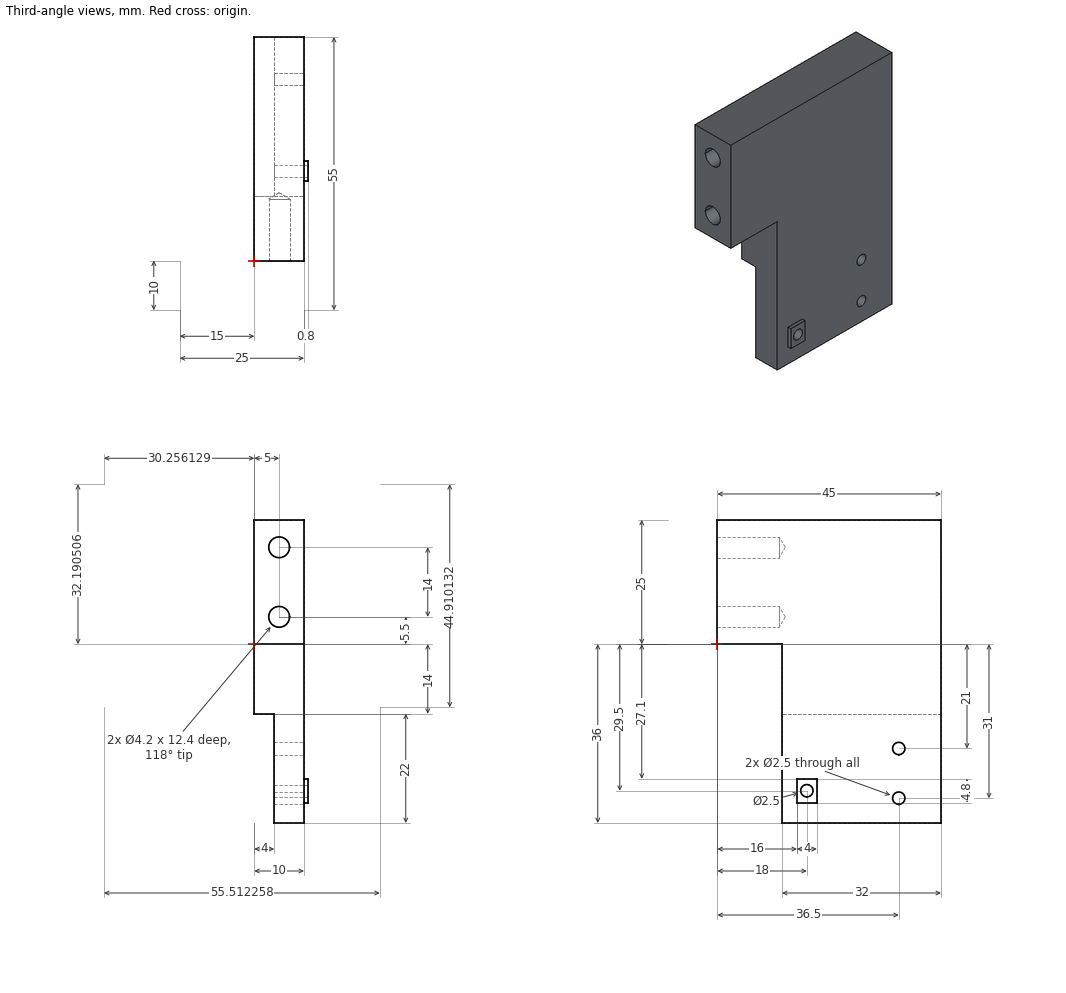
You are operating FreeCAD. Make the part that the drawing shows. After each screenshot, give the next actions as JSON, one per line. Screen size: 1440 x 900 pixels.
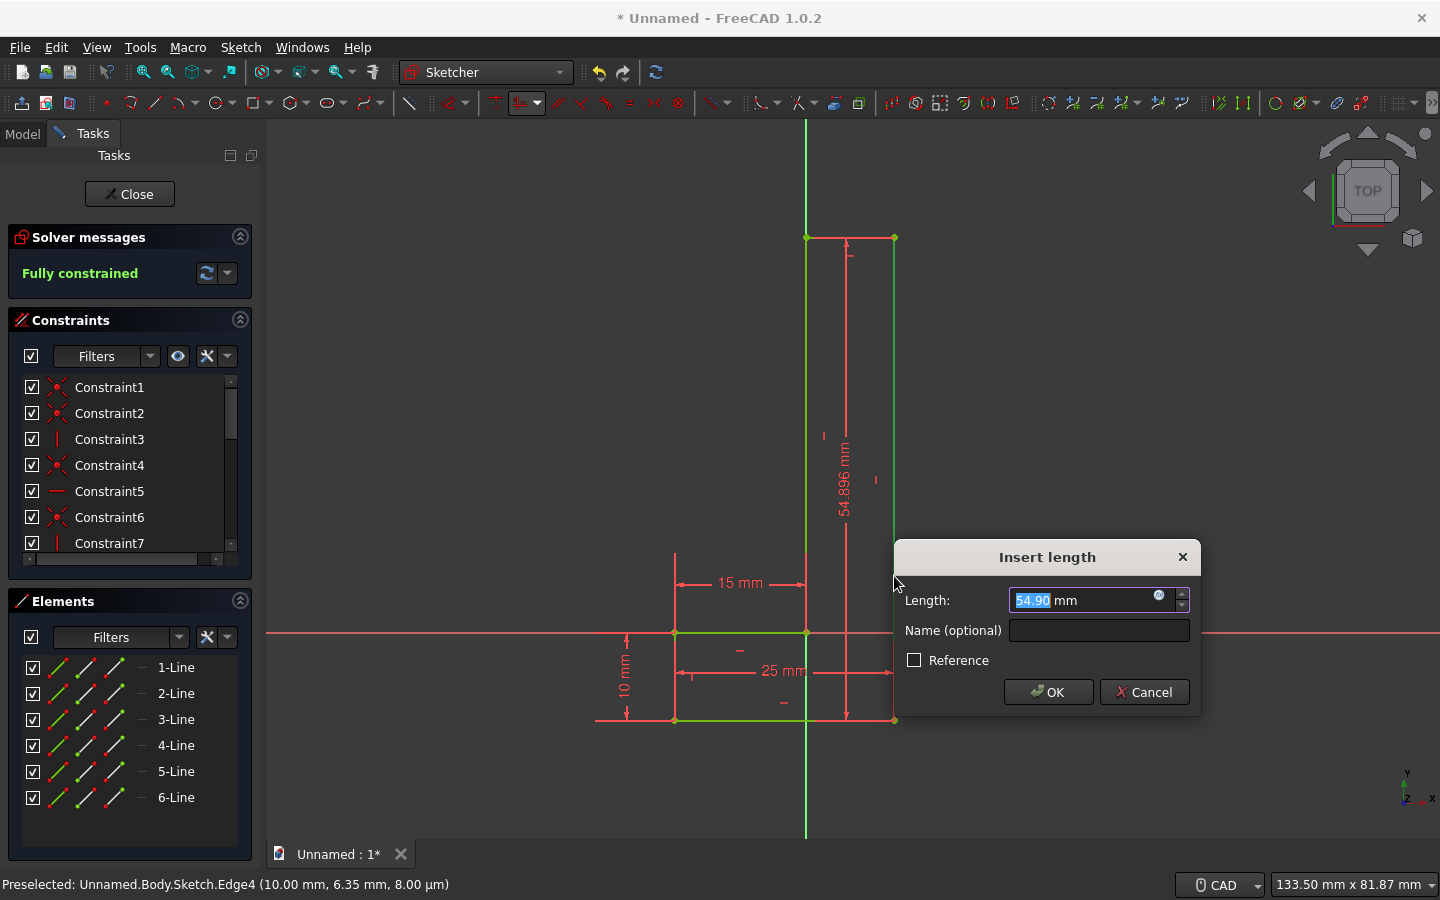
{"action": "type", "text": "55"}
{"action": "key", "text": "Return"}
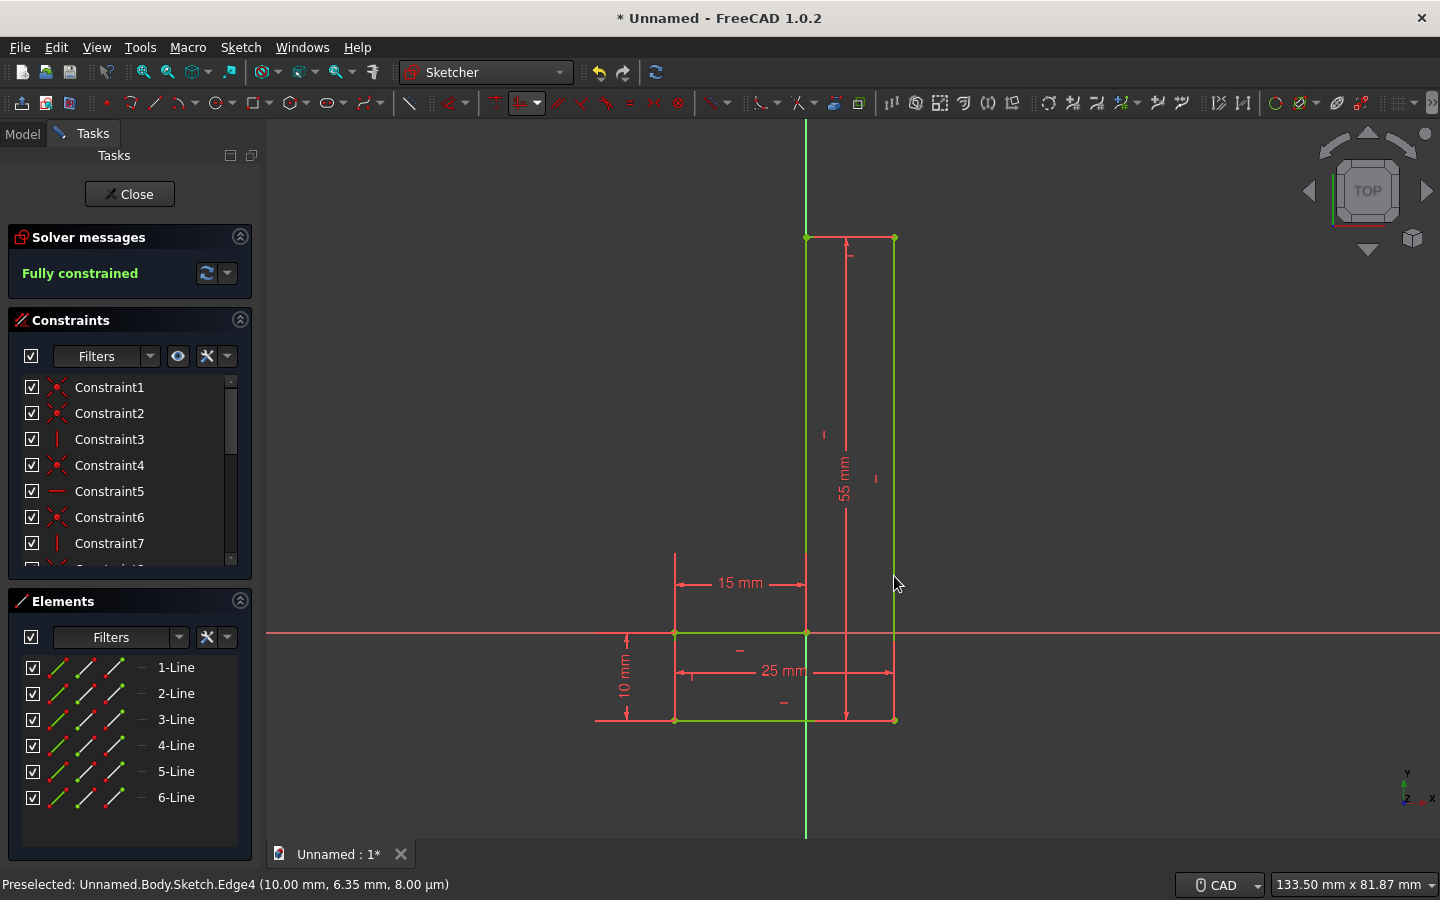
{"action": "left_click", "coordinate": [130, 194]}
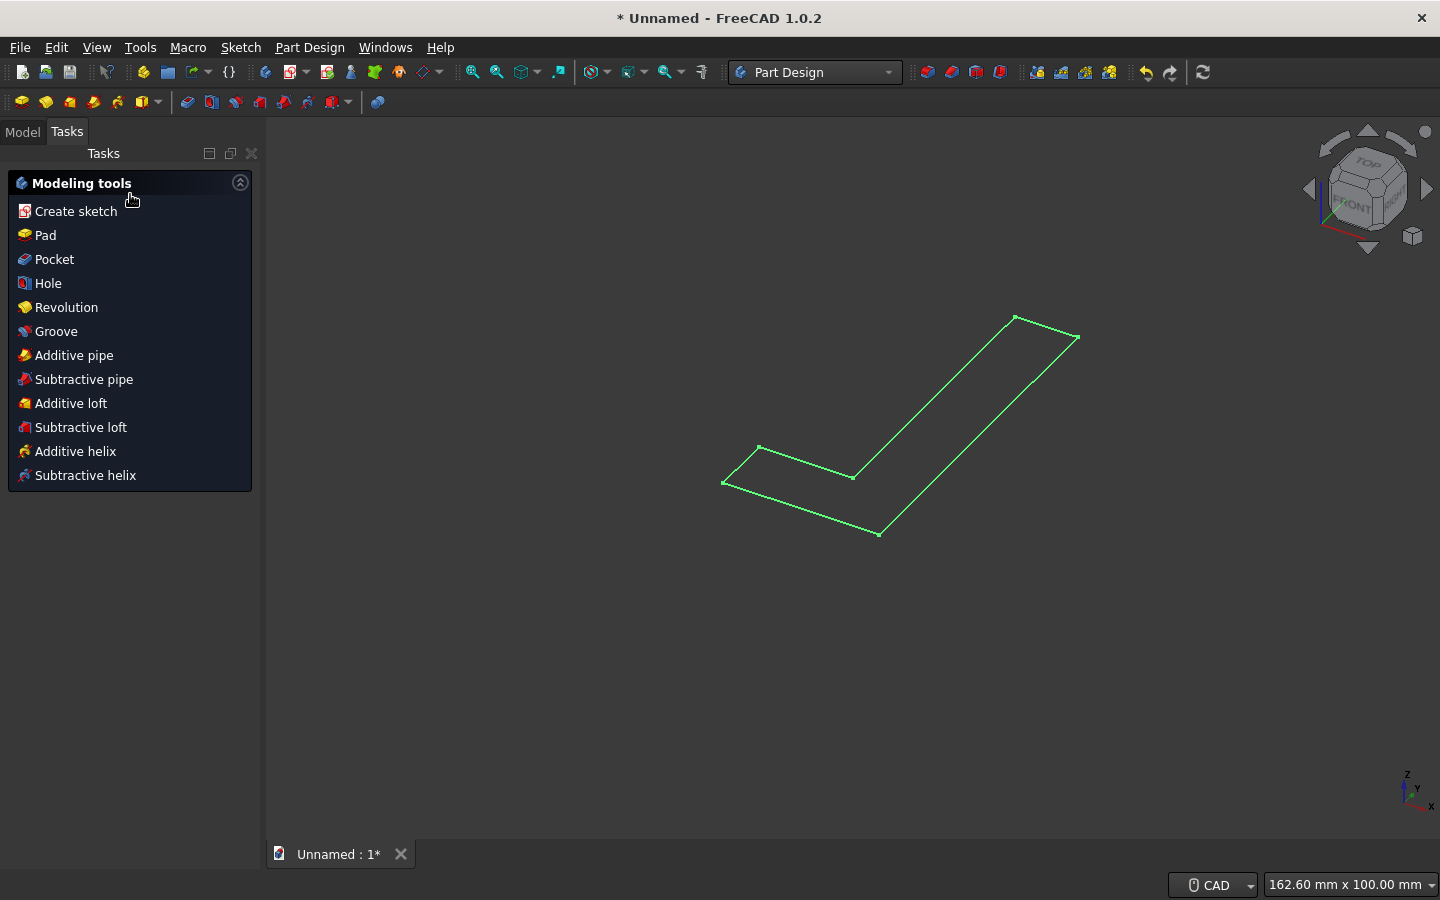
{"action": "left_click", "coordinate": [22, 102]}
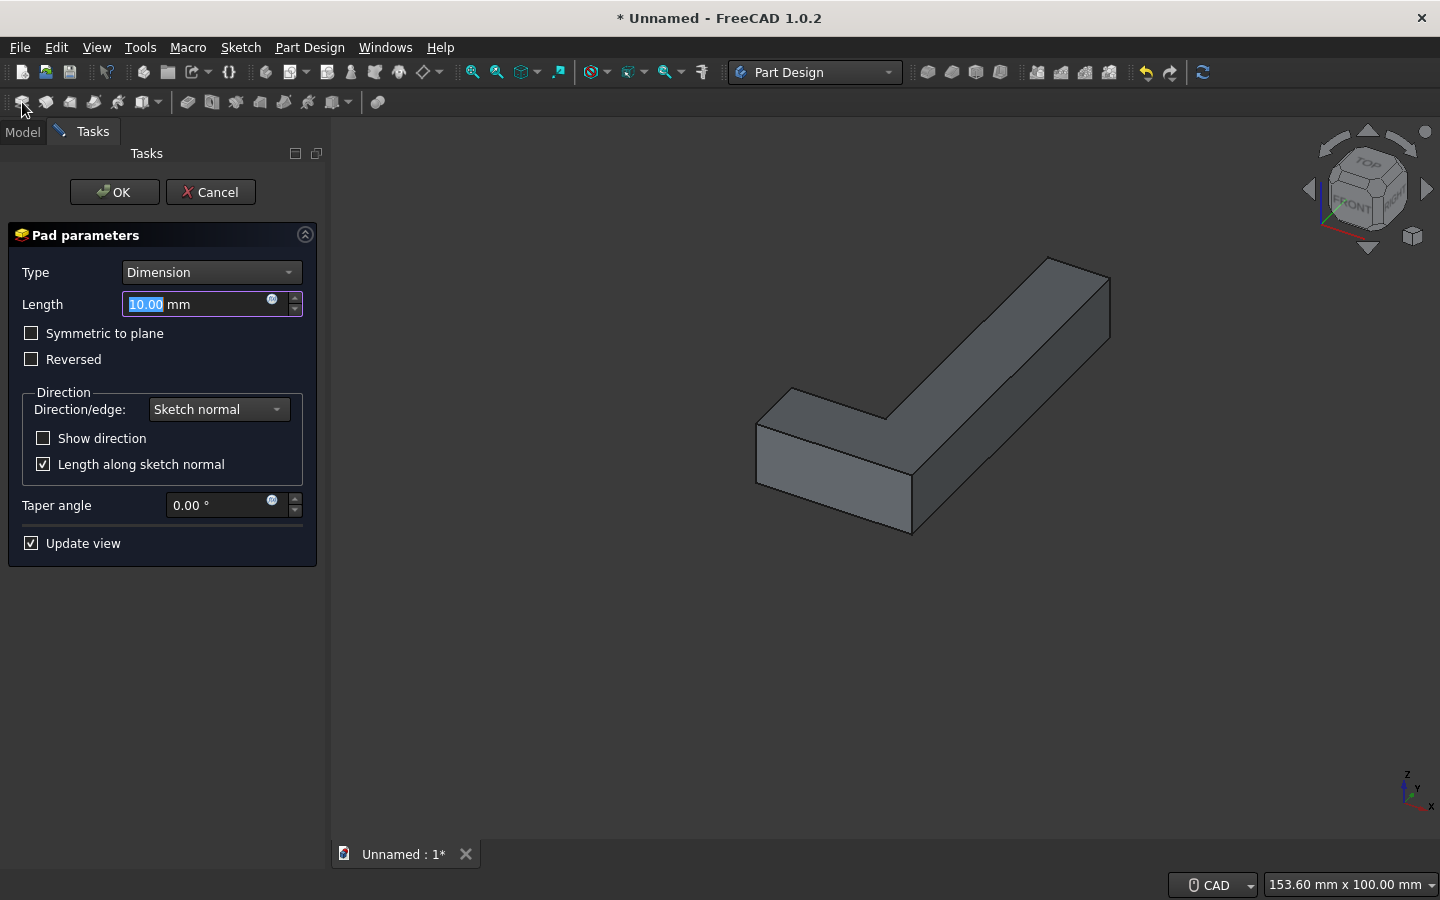
{"action": "type", "text": "25"}
{"action": "key", "text": "Tab"}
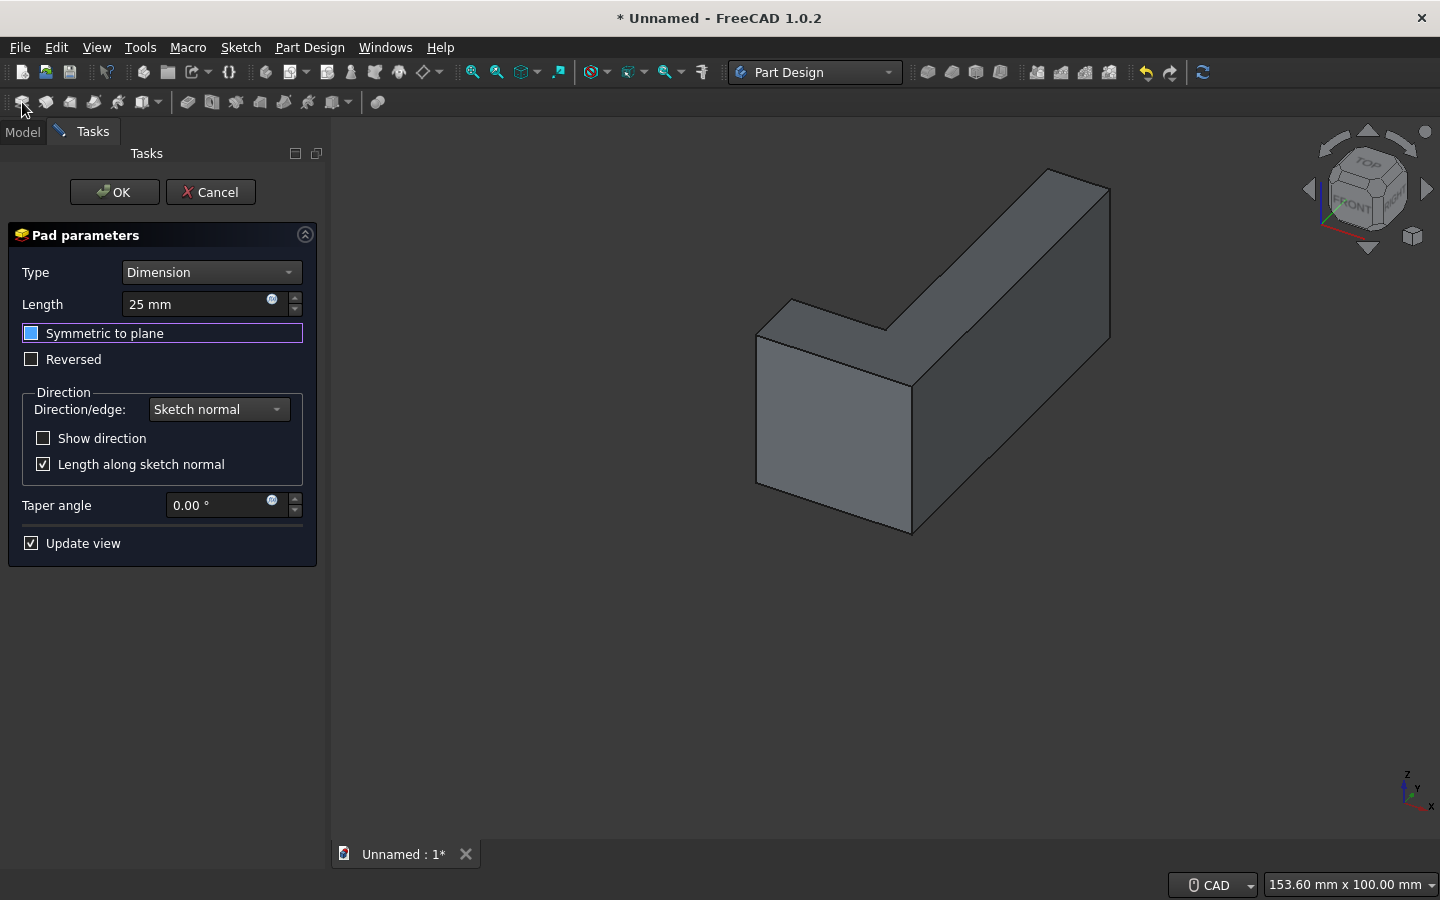
{"action": "left_click", "coordinate": [115, 192]}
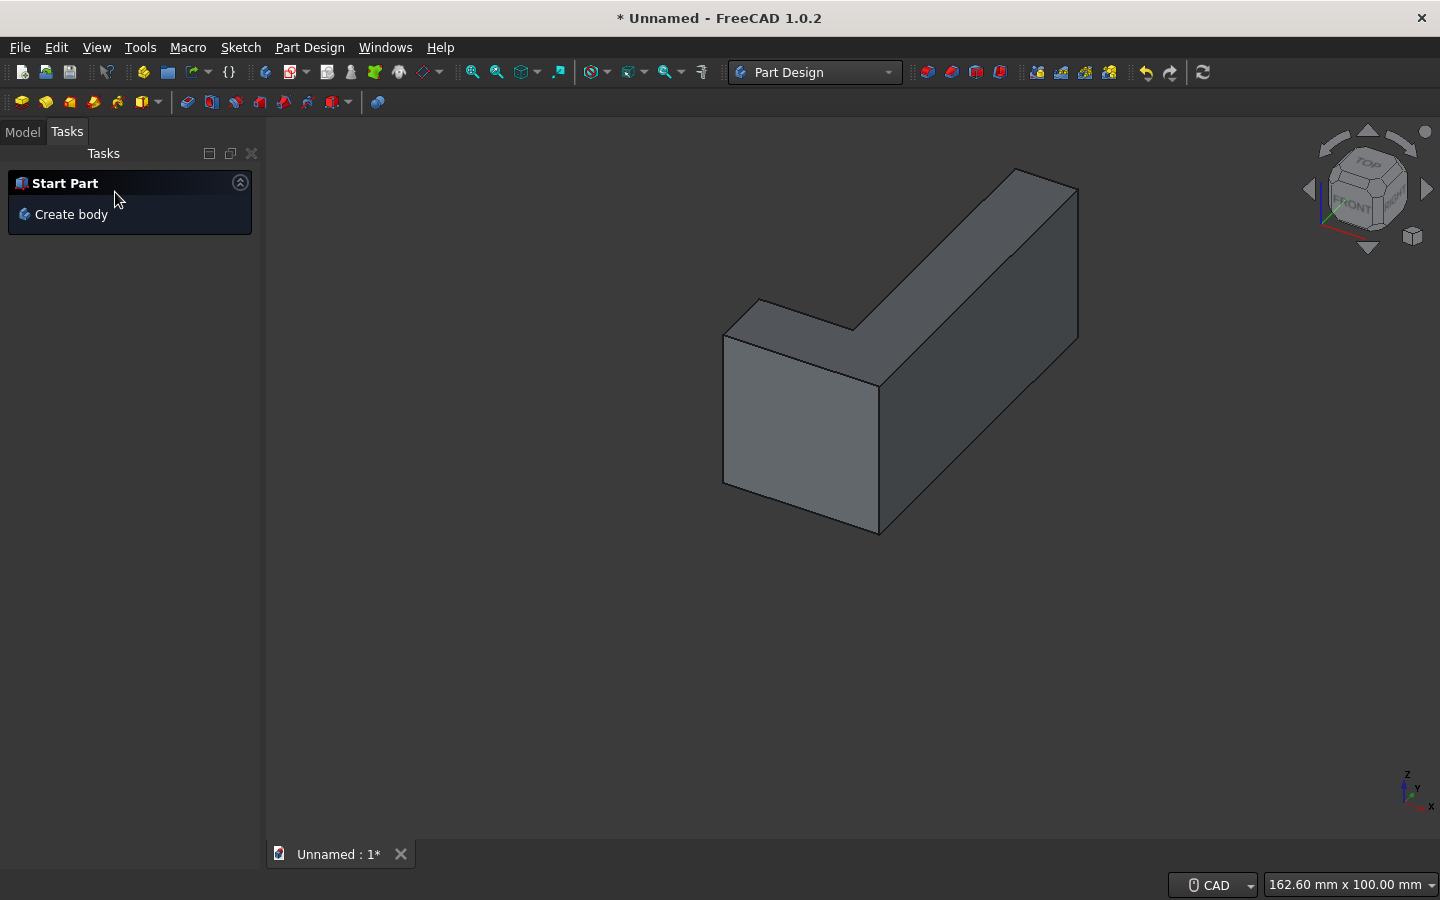
{"action": "key", "text": "6"}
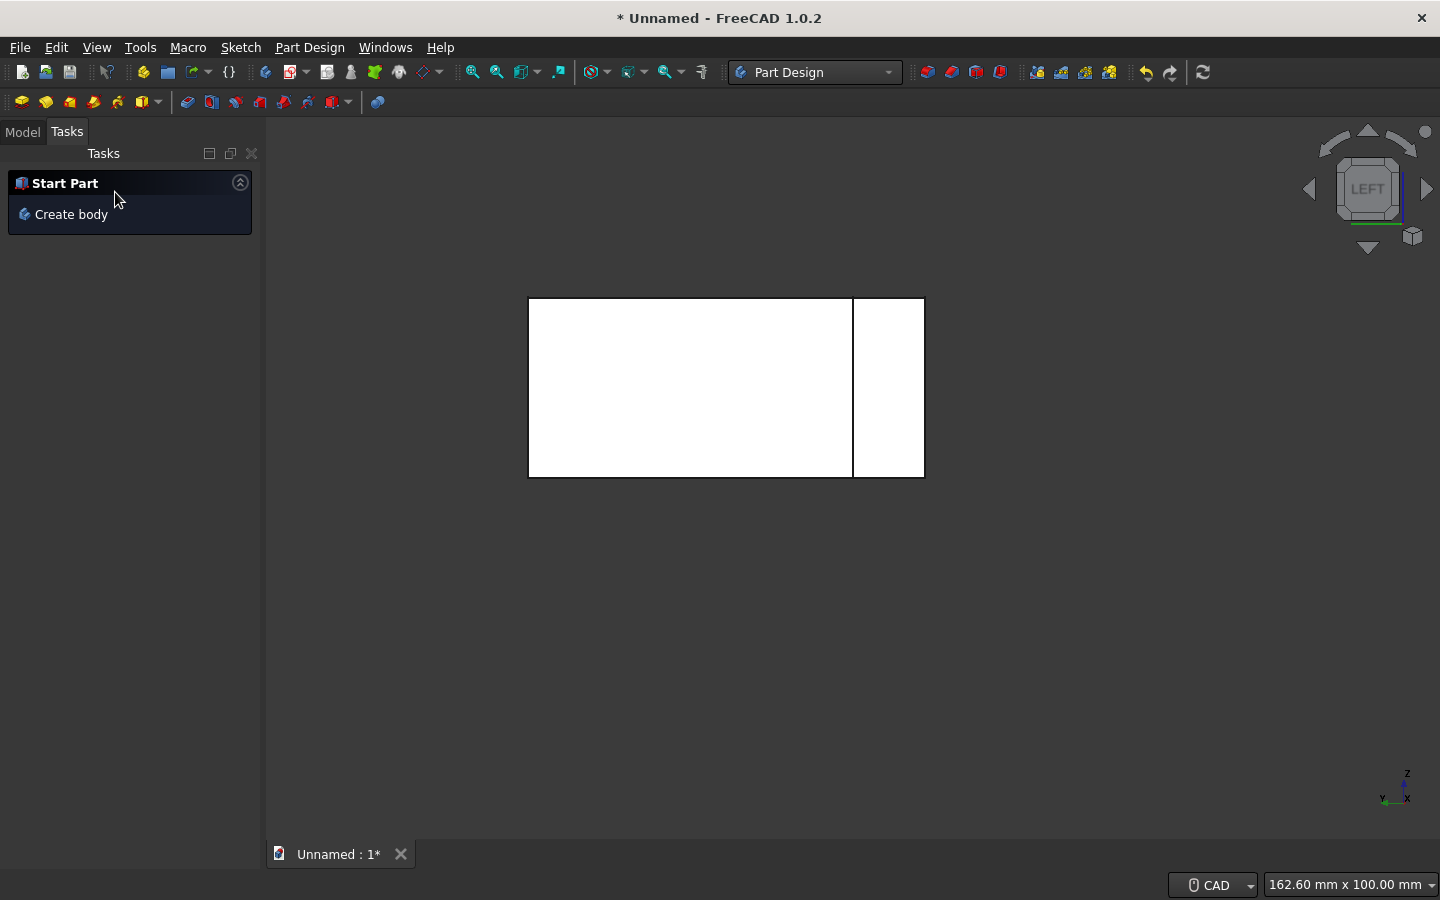
{"action": "key", "text": "v f"}